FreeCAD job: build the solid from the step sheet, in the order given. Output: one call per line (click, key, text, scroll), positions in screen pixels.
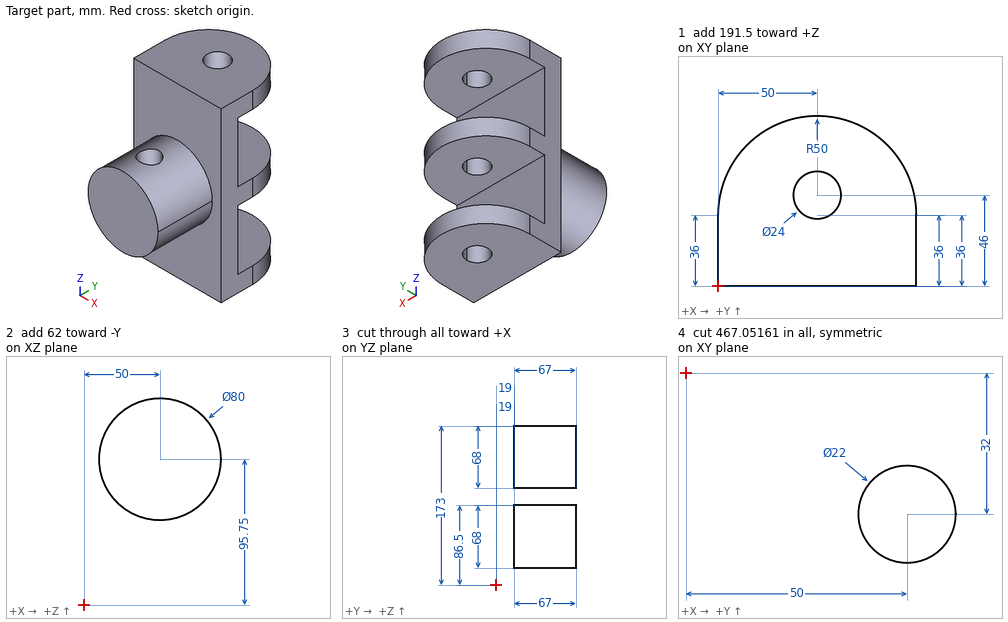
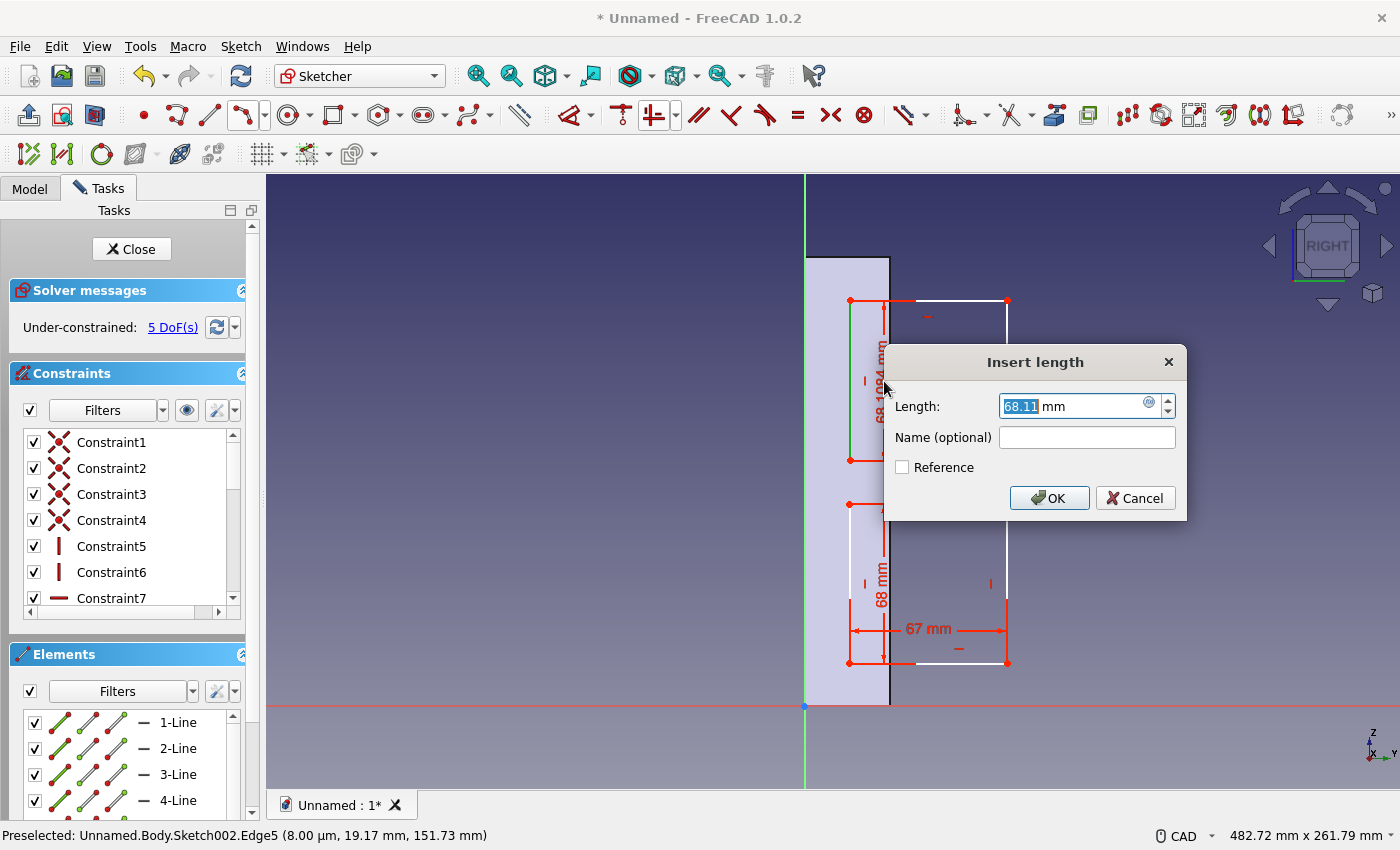
text(68)
key(Return)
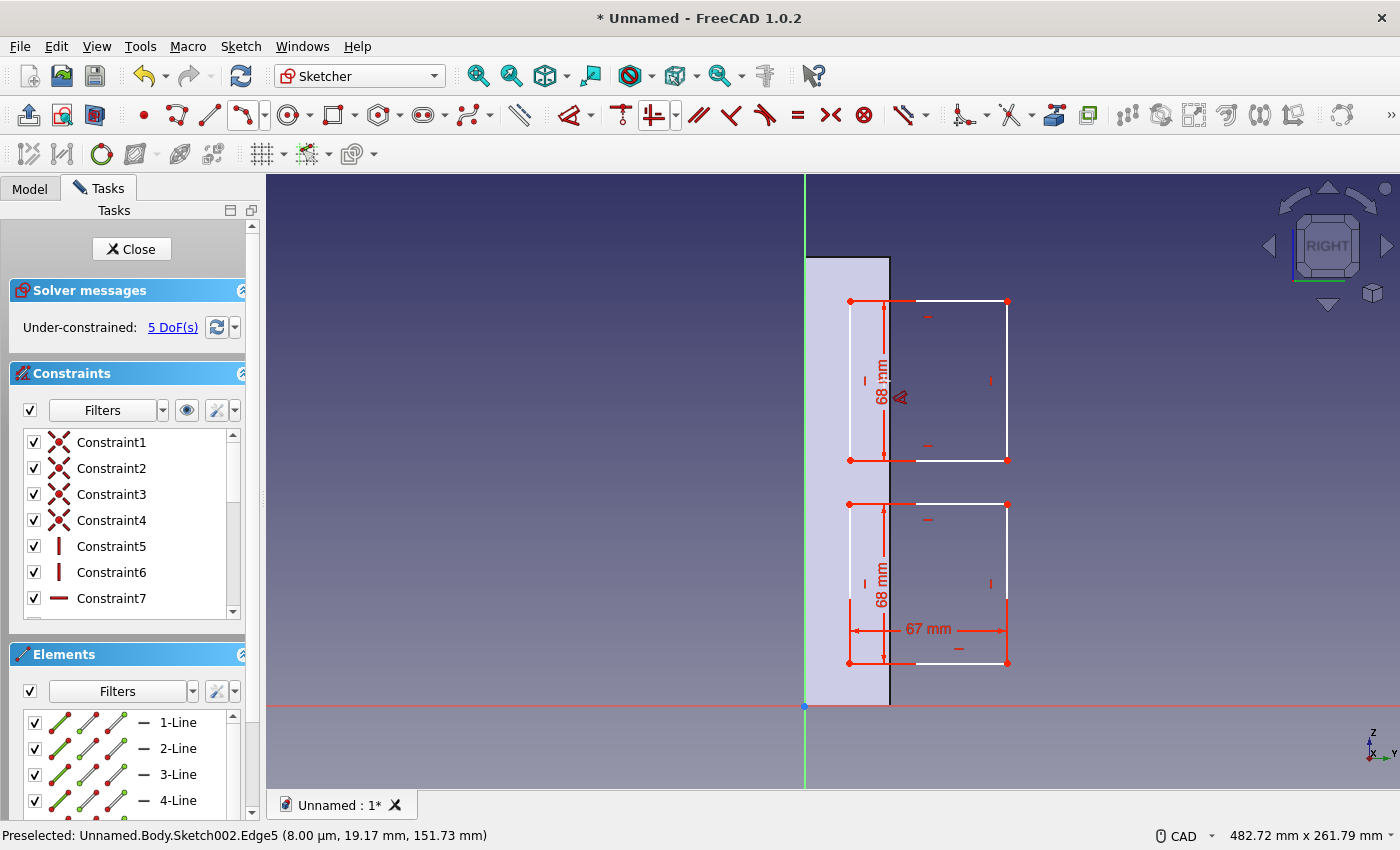
click(897, 461)
click(929, 427)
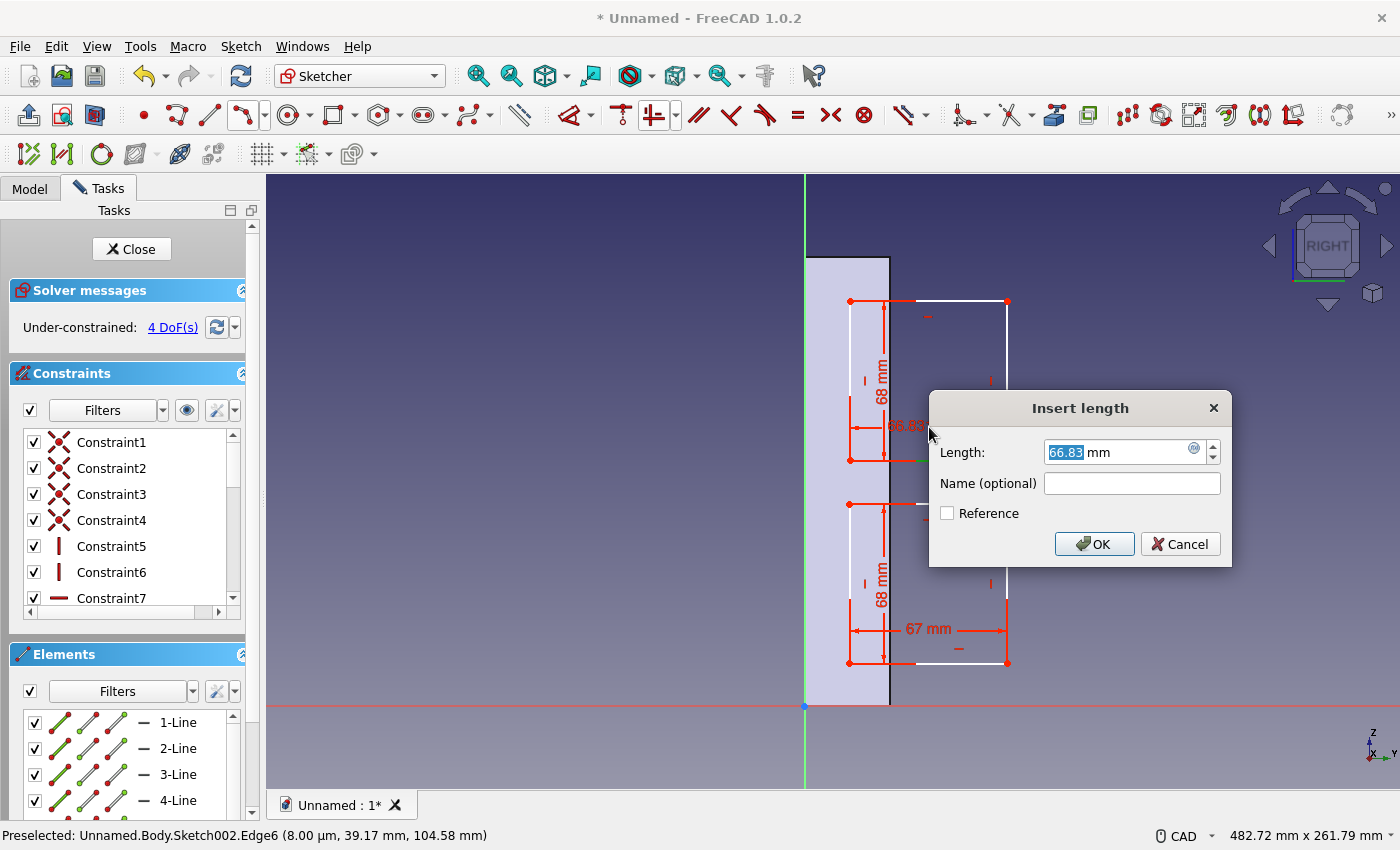
text(67)
key(Return)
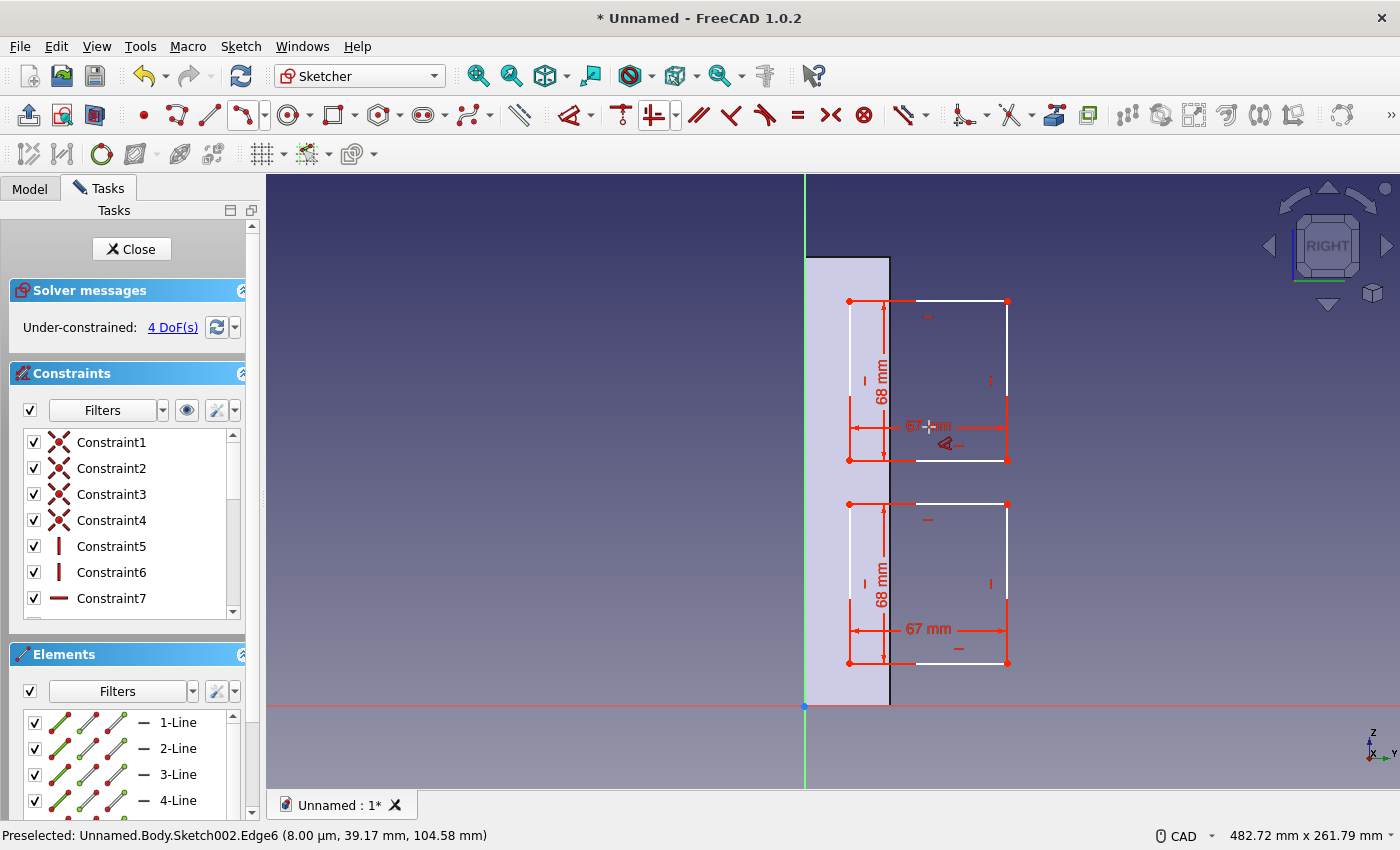
click(850, 504)
click(827, 740)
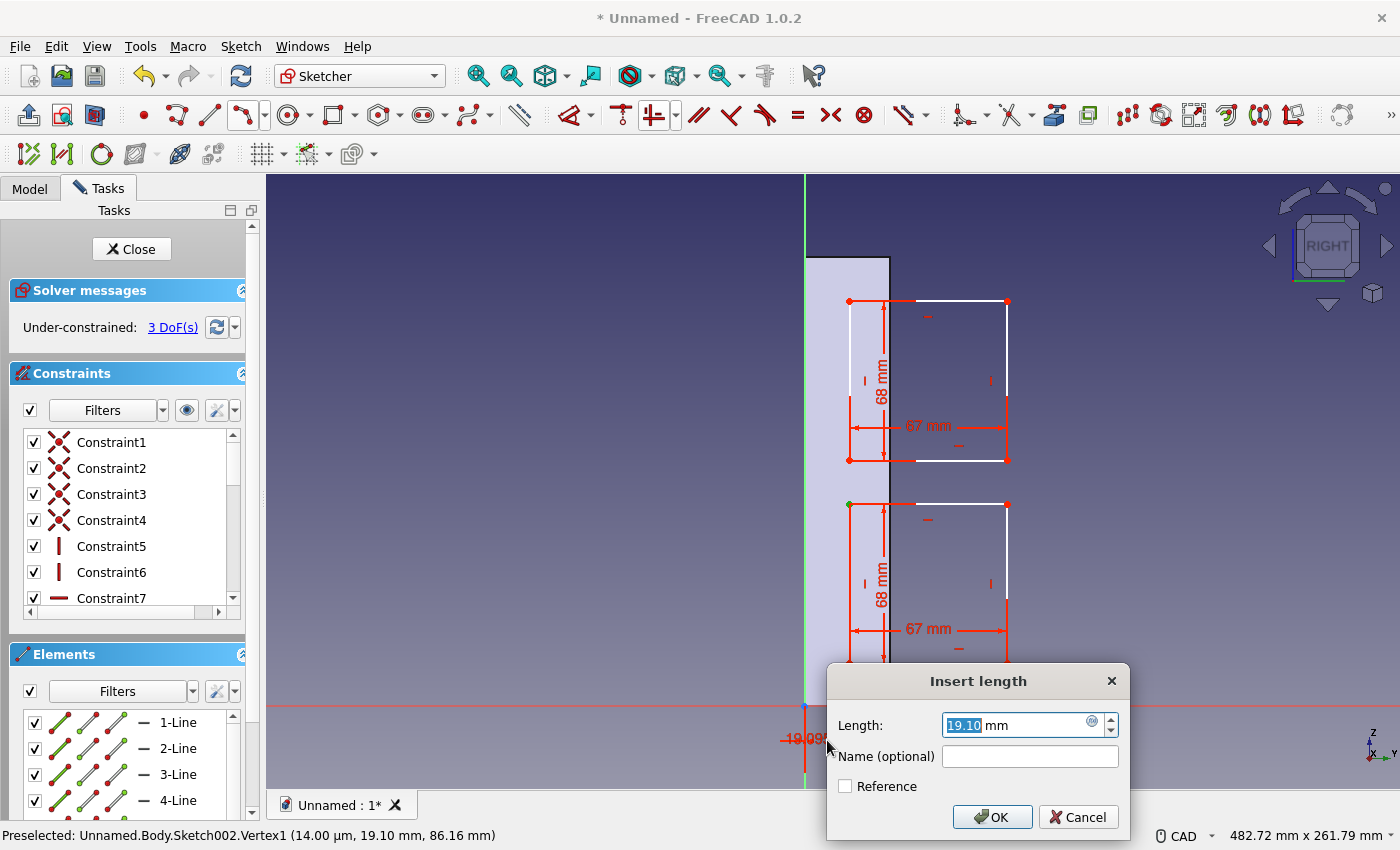
text(19)
key(Return)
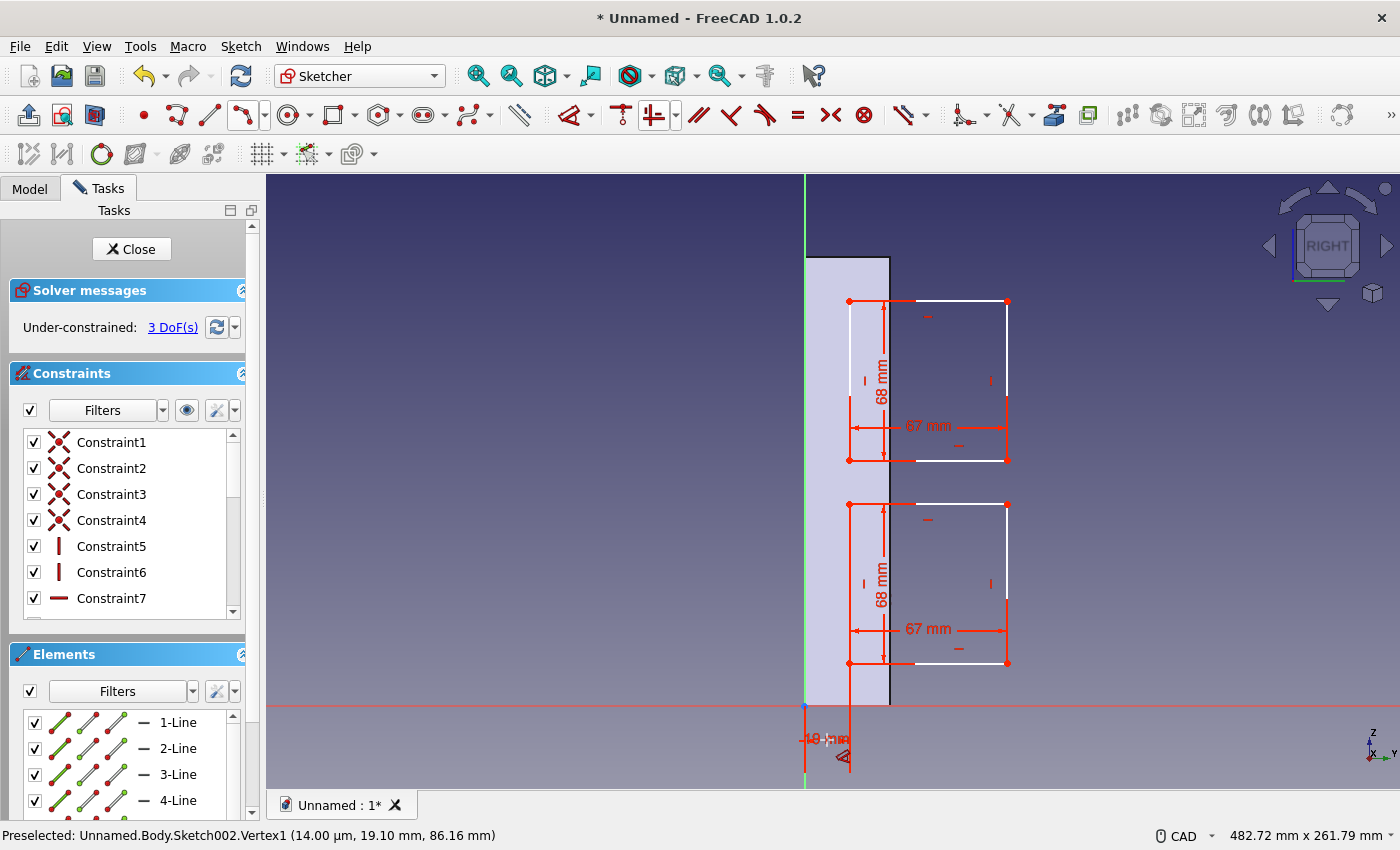
click(850, 301)
click(827, 267)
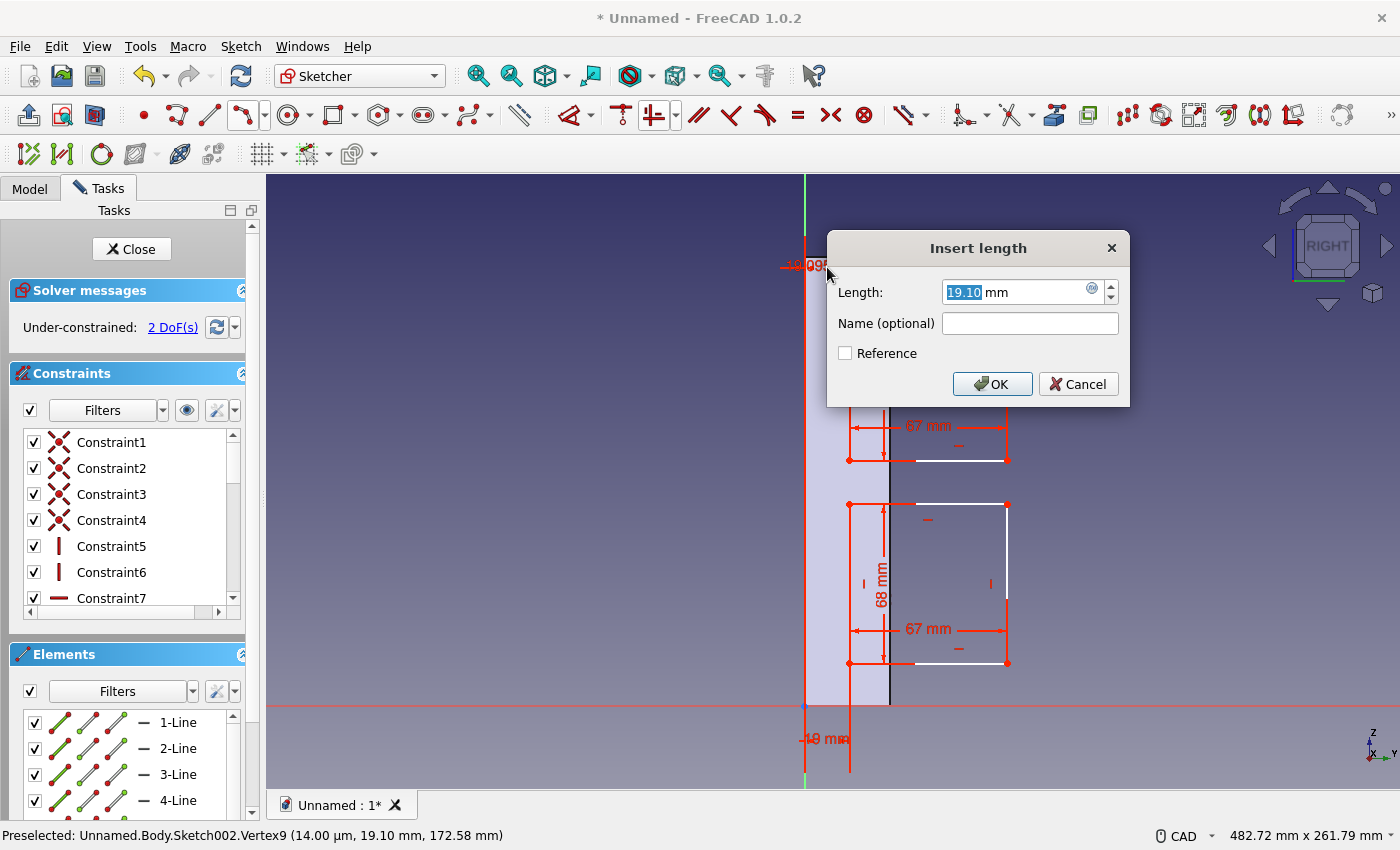
text(19)
key(Return)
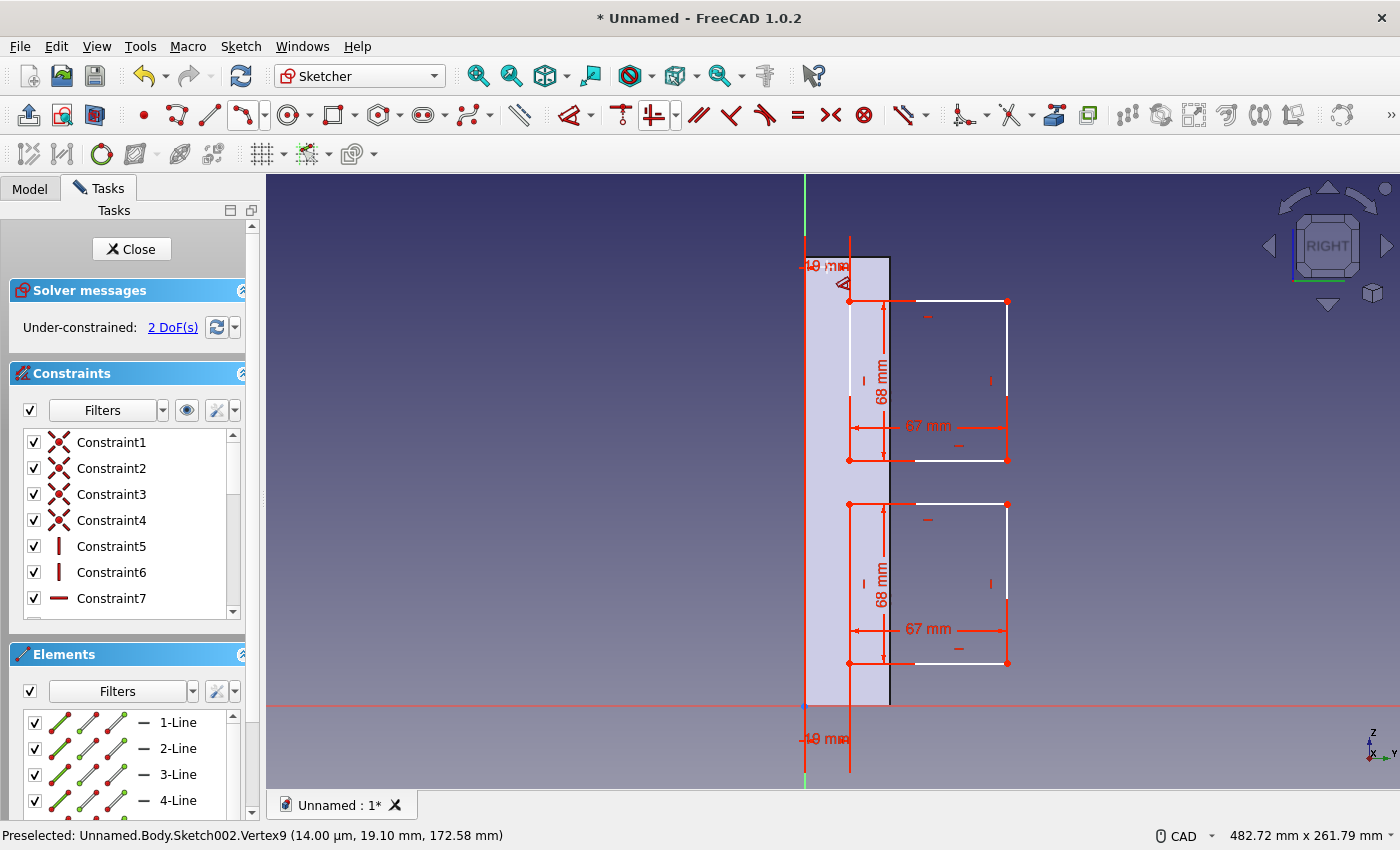
click(850, 301)
click(771, 504)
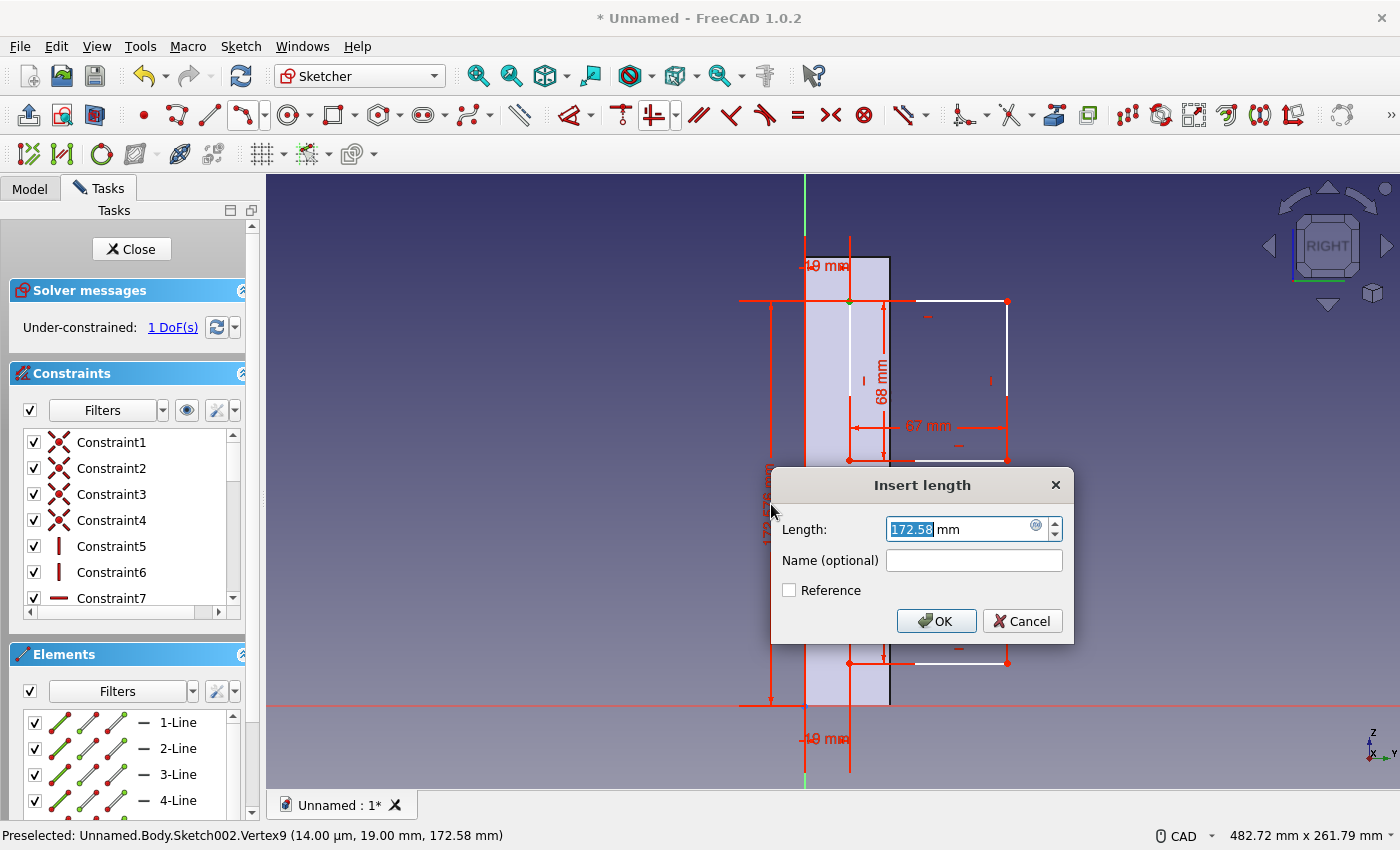
text(173)
key(Return)